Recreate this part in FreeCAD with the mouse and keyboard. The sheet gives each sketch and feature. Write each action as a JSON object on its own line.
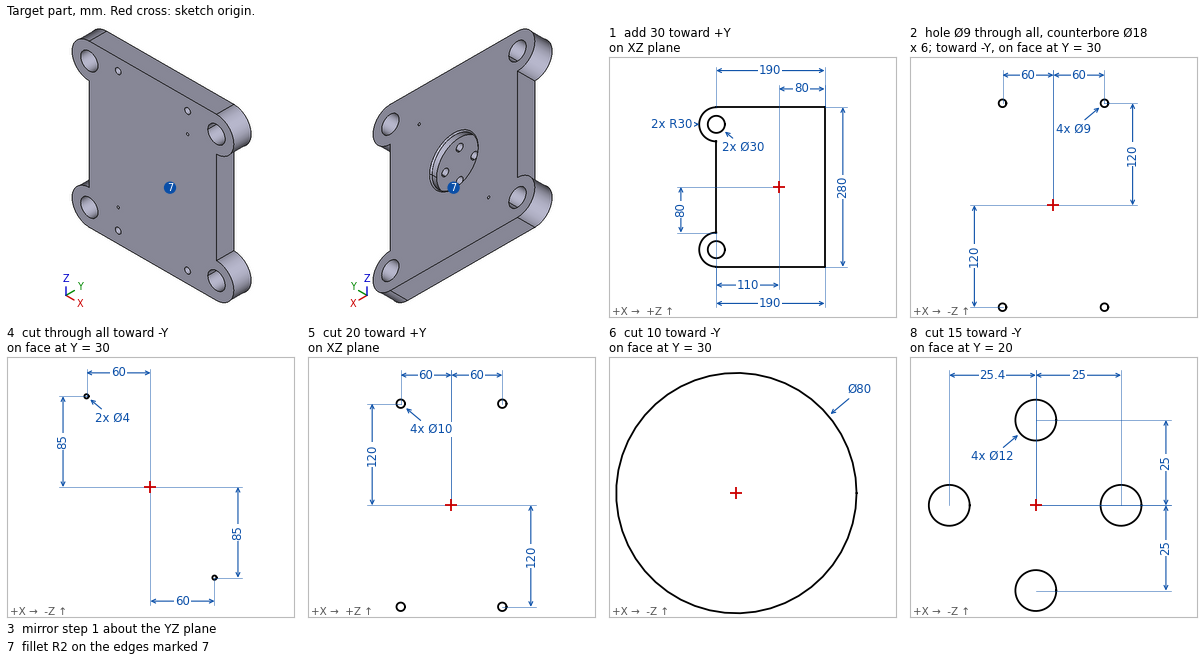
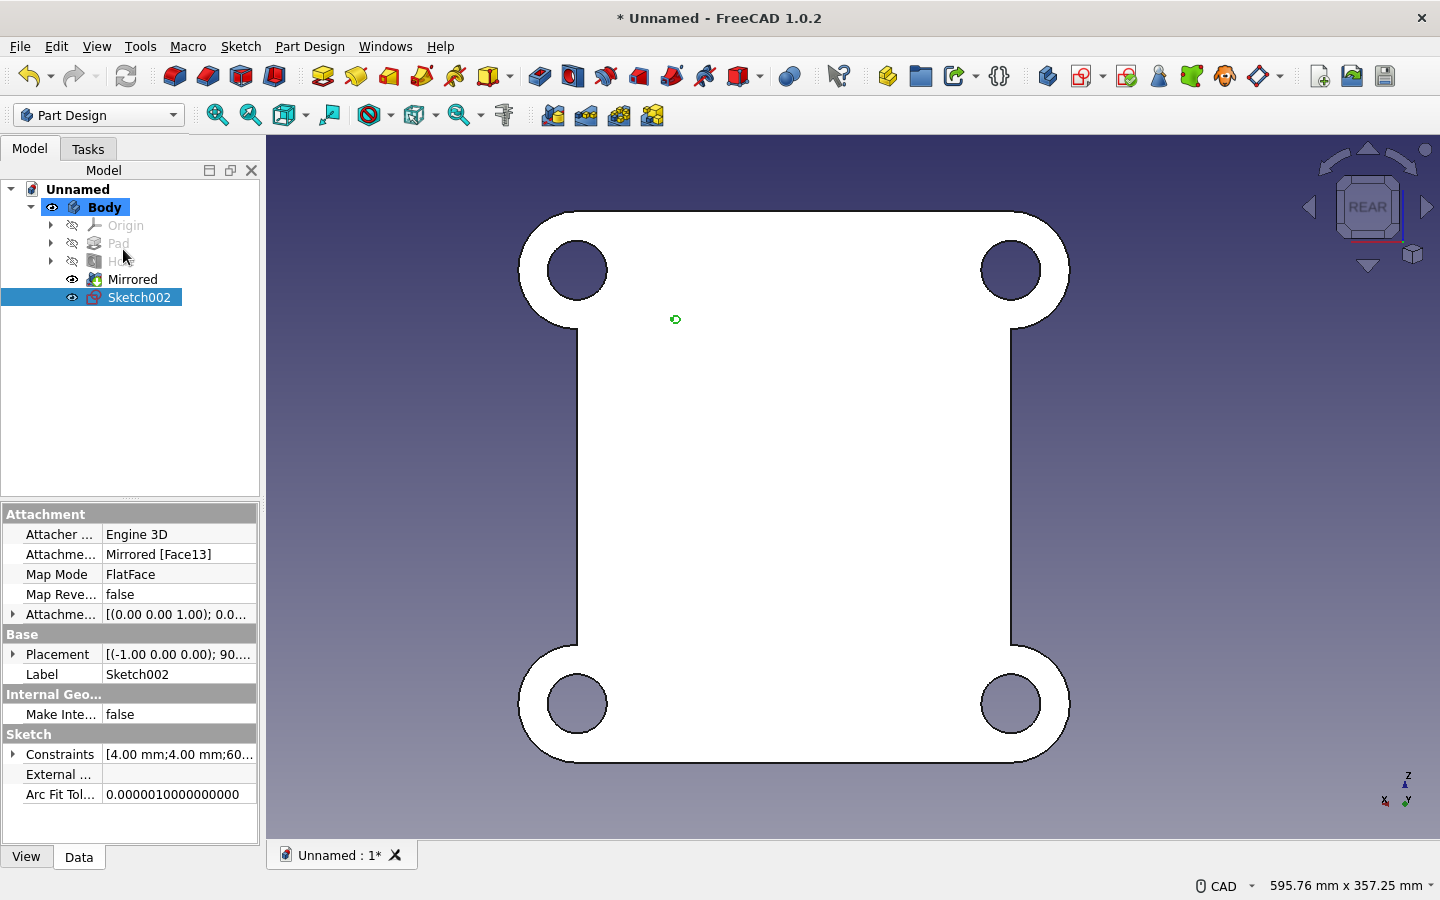
{"action": "left_click", "coordinate": [540, 76]}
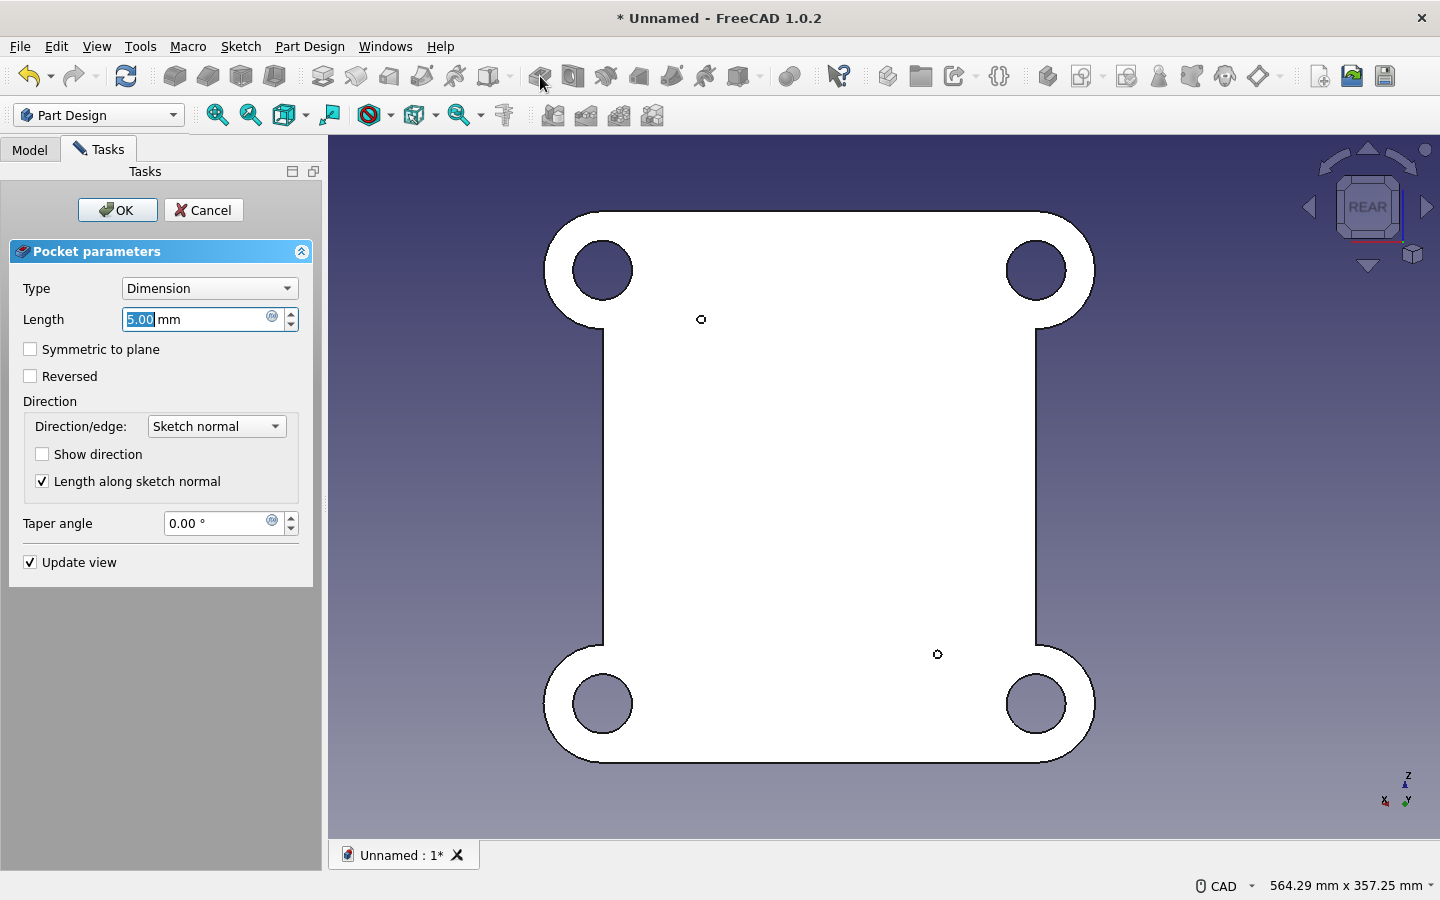
{"action": "left_click", "coordinate": [210, 288]}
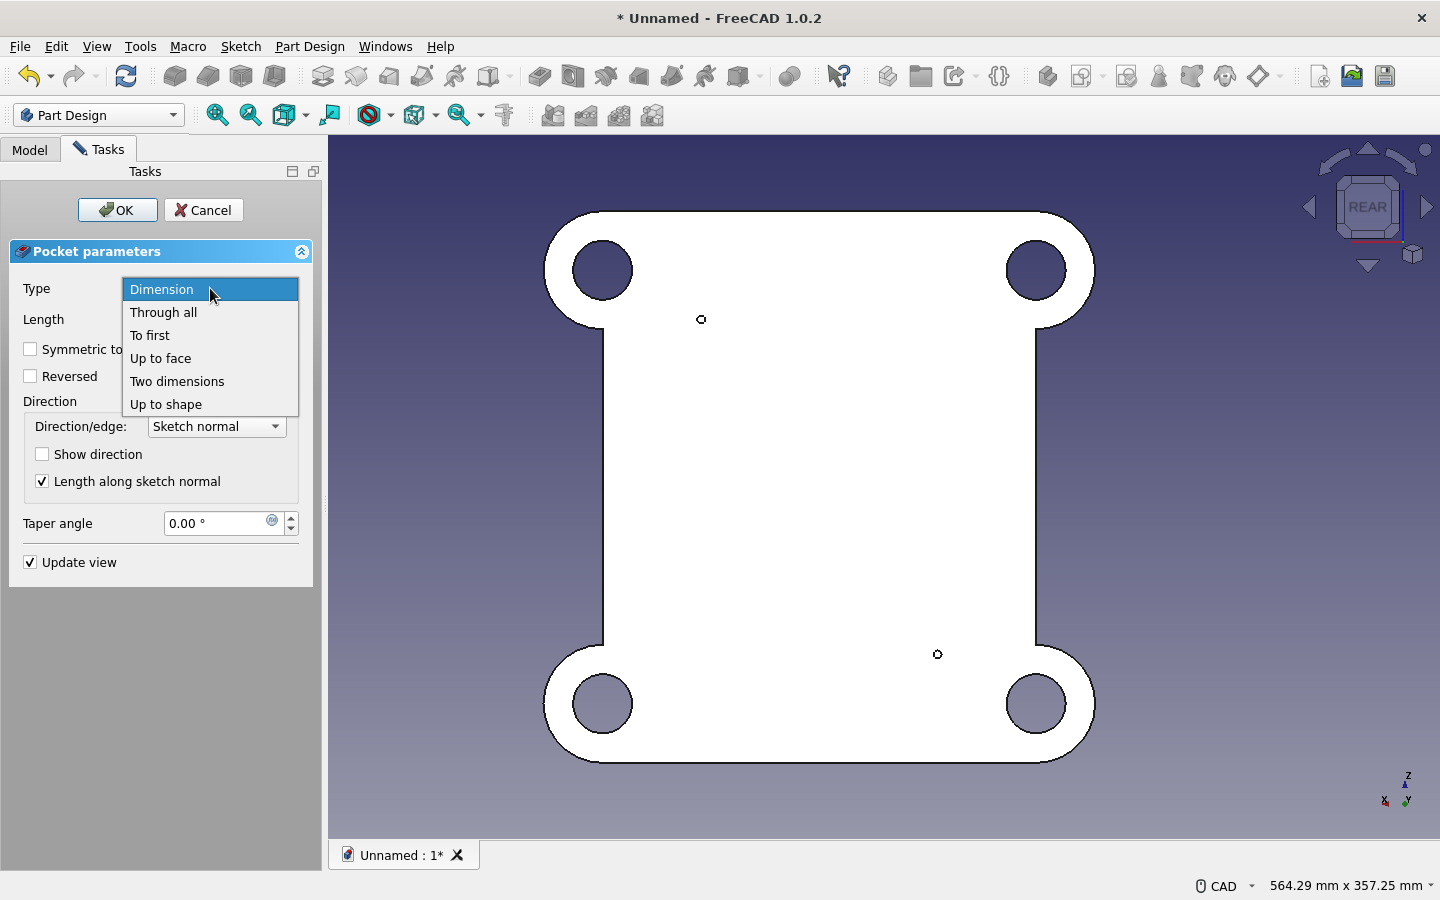
{"action": "left_click", "coordinate": [208, 312]}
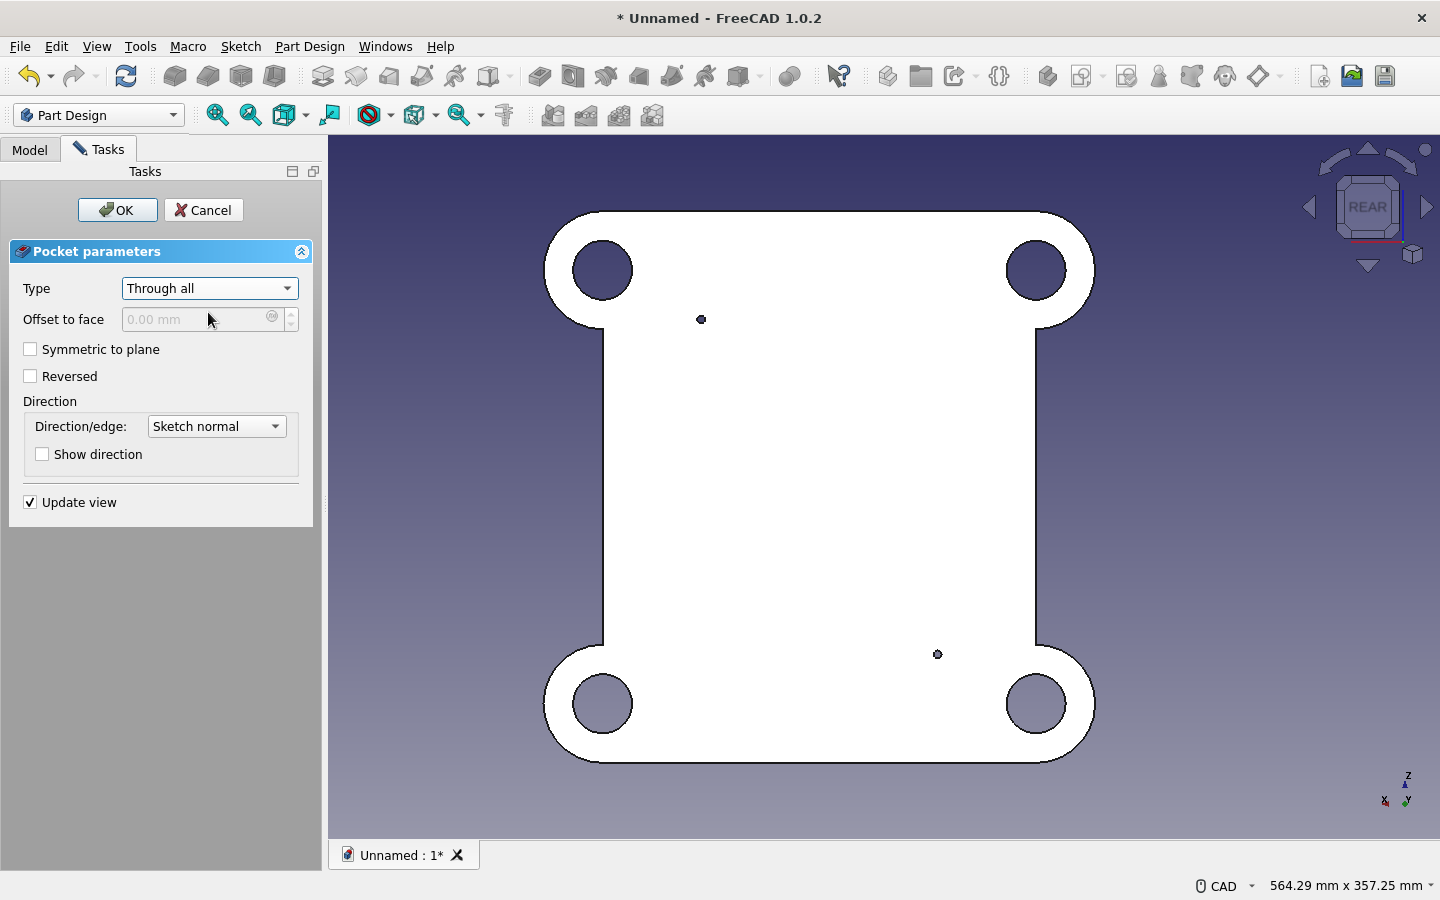
{"action": "left_click", "coordinate": [118, 210]}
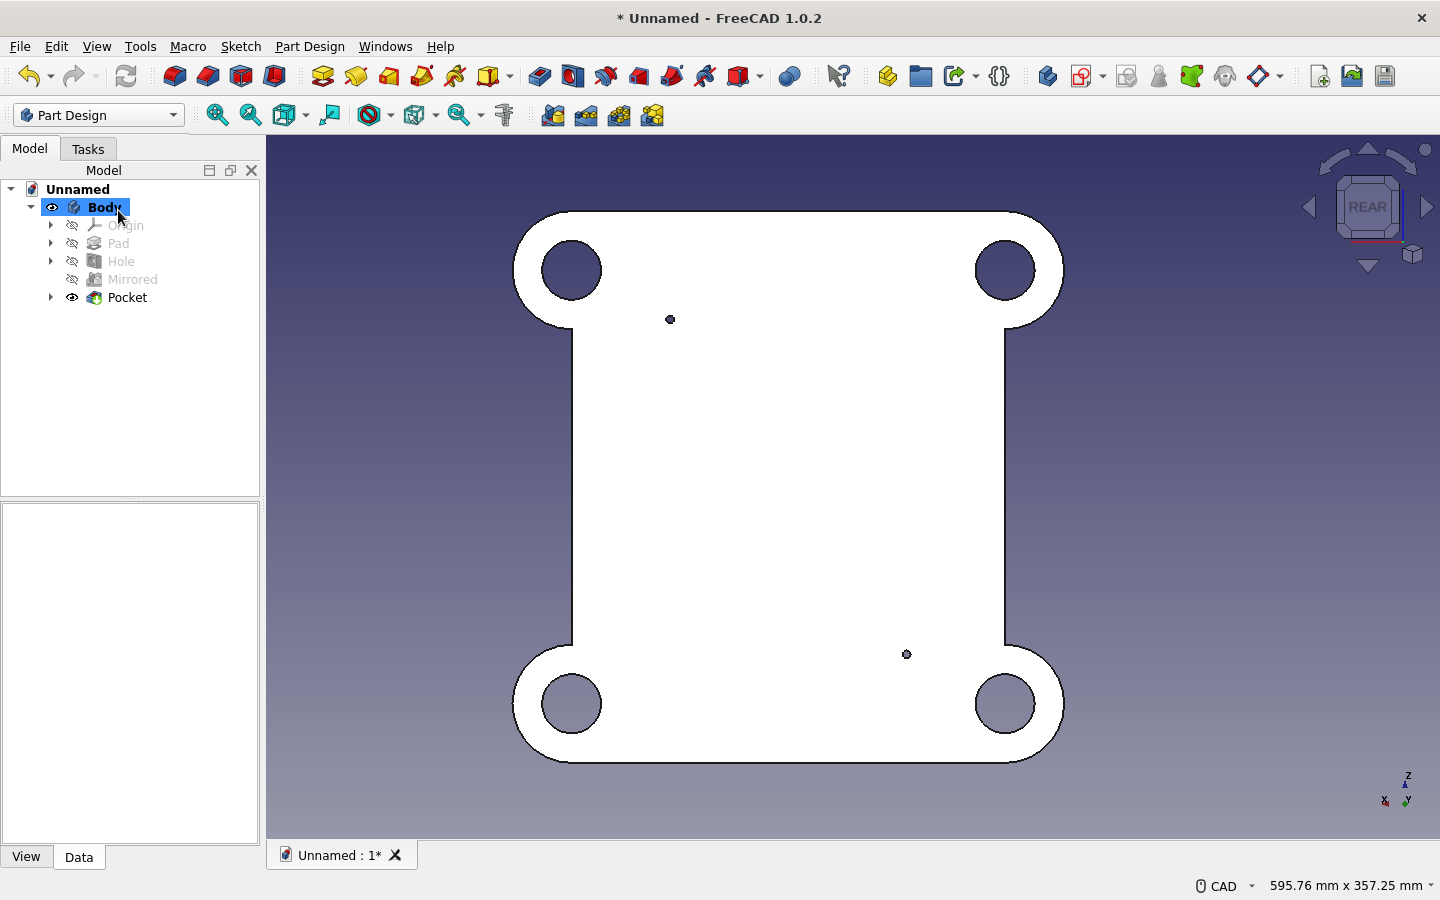
{"action": "left_click", "coordinate": [1080, 76]}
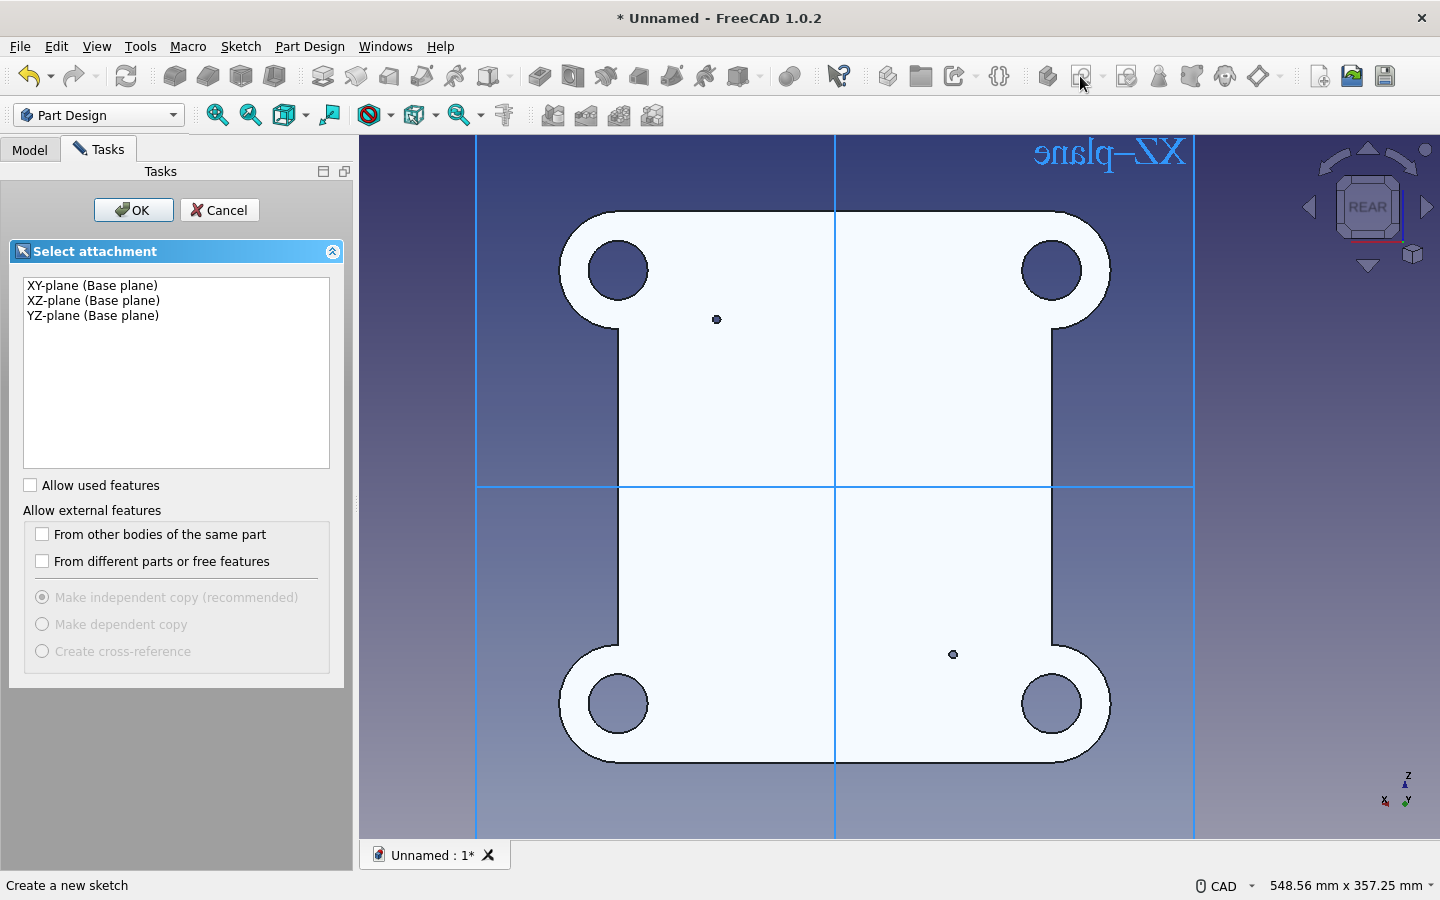
{"action": "left_click", "coordinate": [84, 300]}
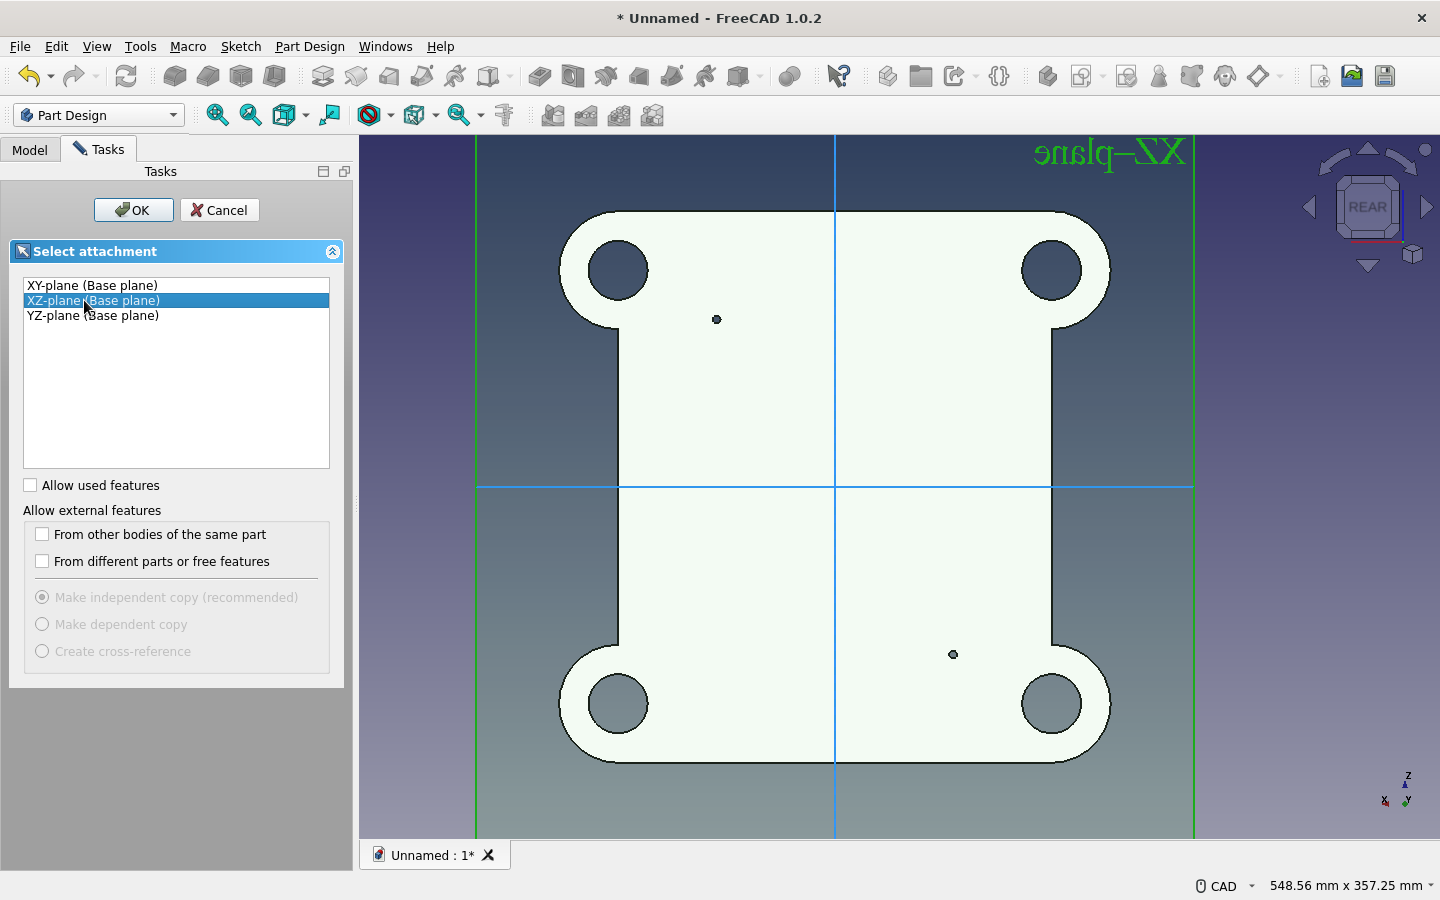
{"action": "left_click", "coordinate": [134, 210]}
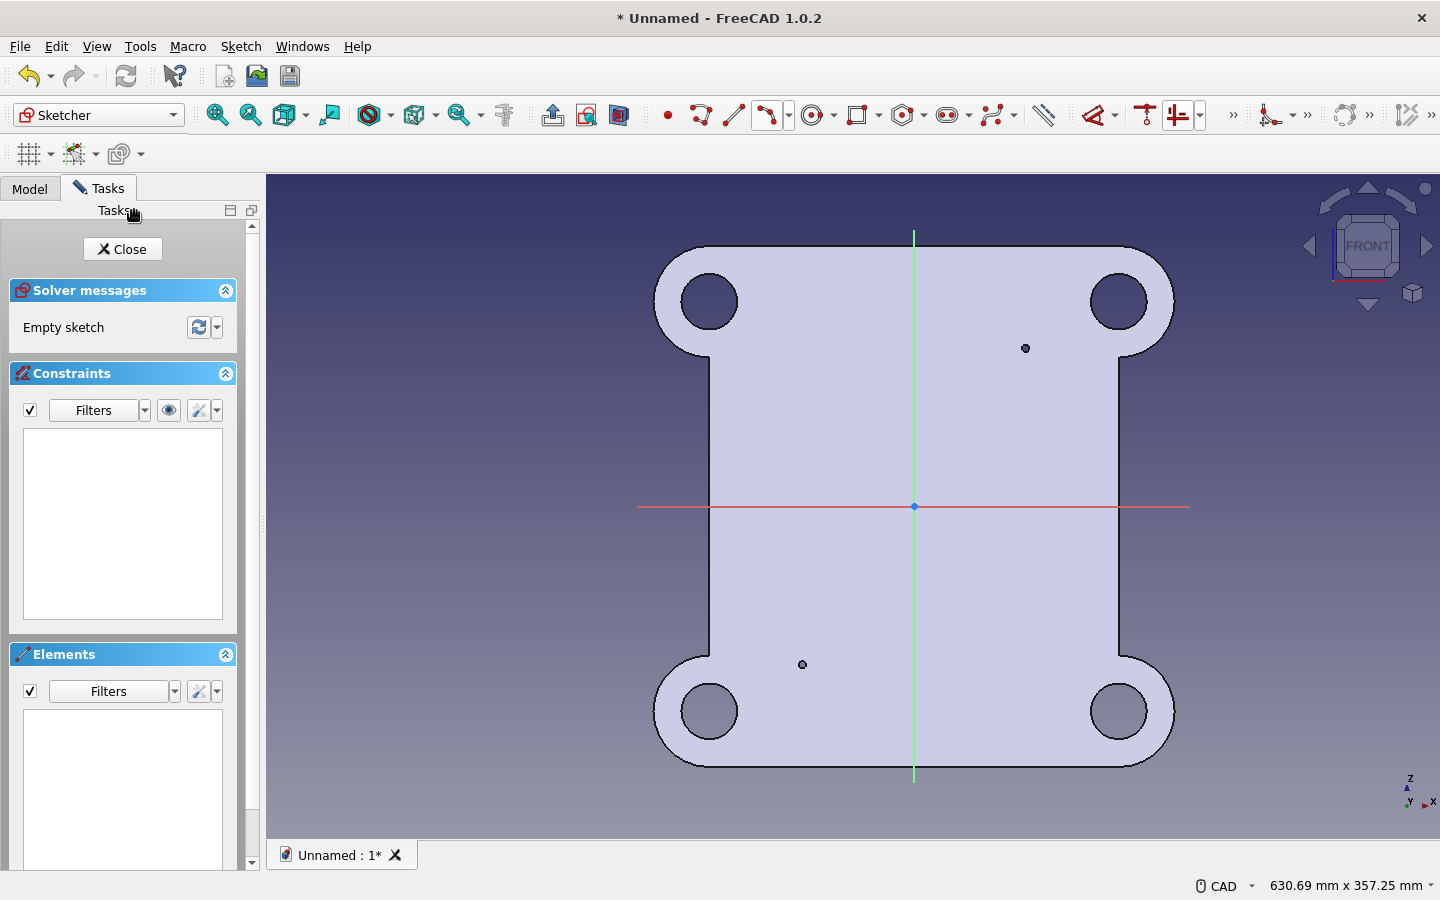
{"action": "left_click", "coordinate": [812, 116]}